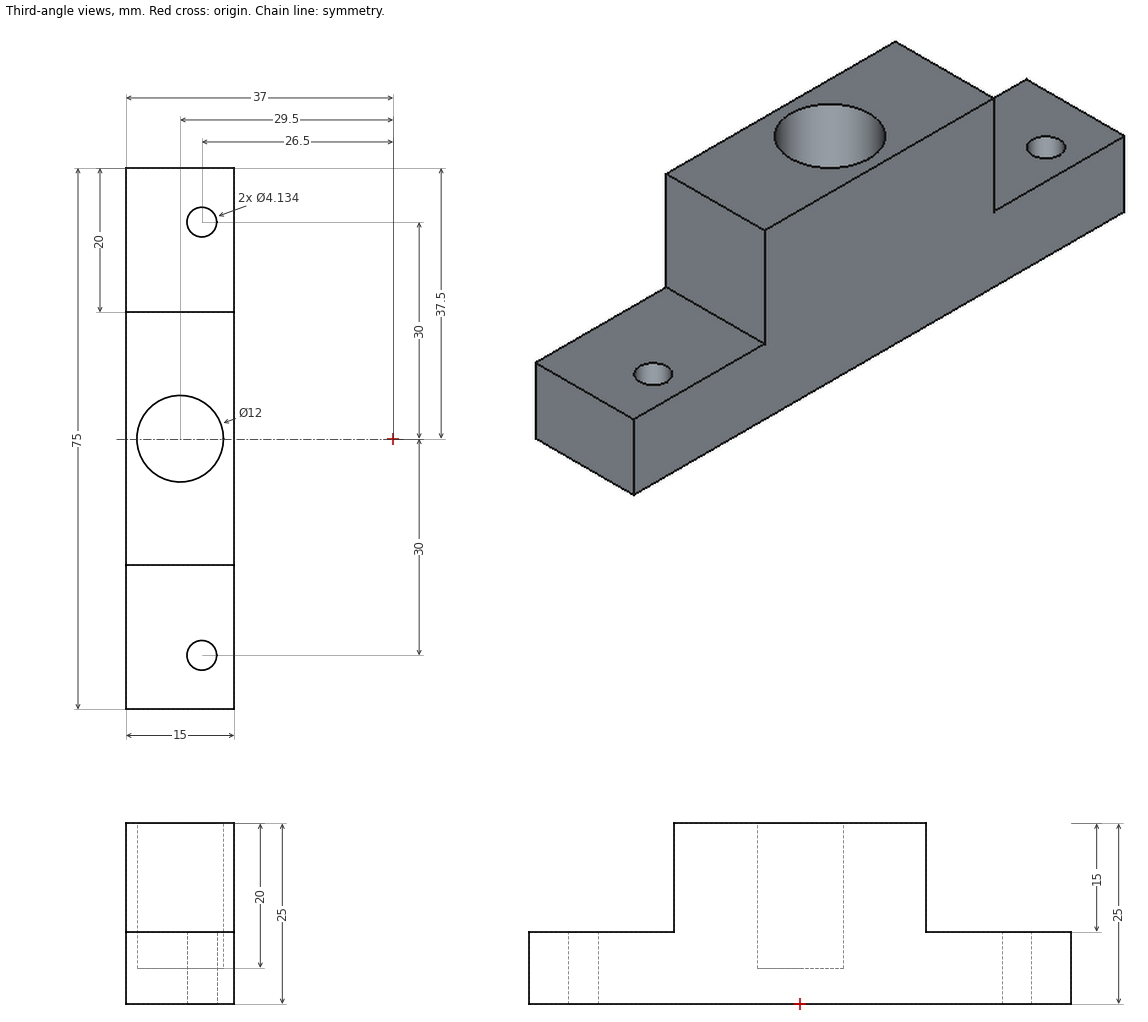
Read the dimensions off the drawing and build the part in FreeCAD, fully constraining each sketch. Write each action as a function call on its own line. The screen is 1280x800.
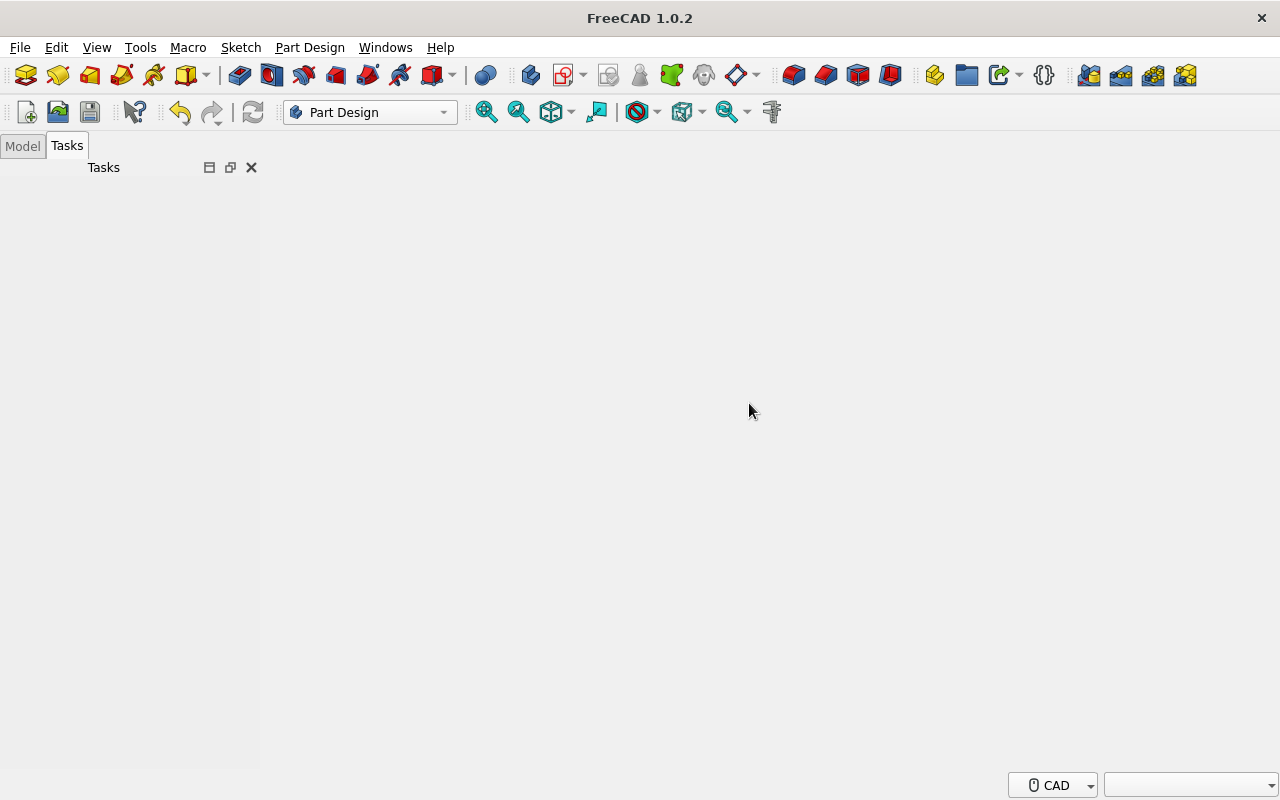
click(26, 112)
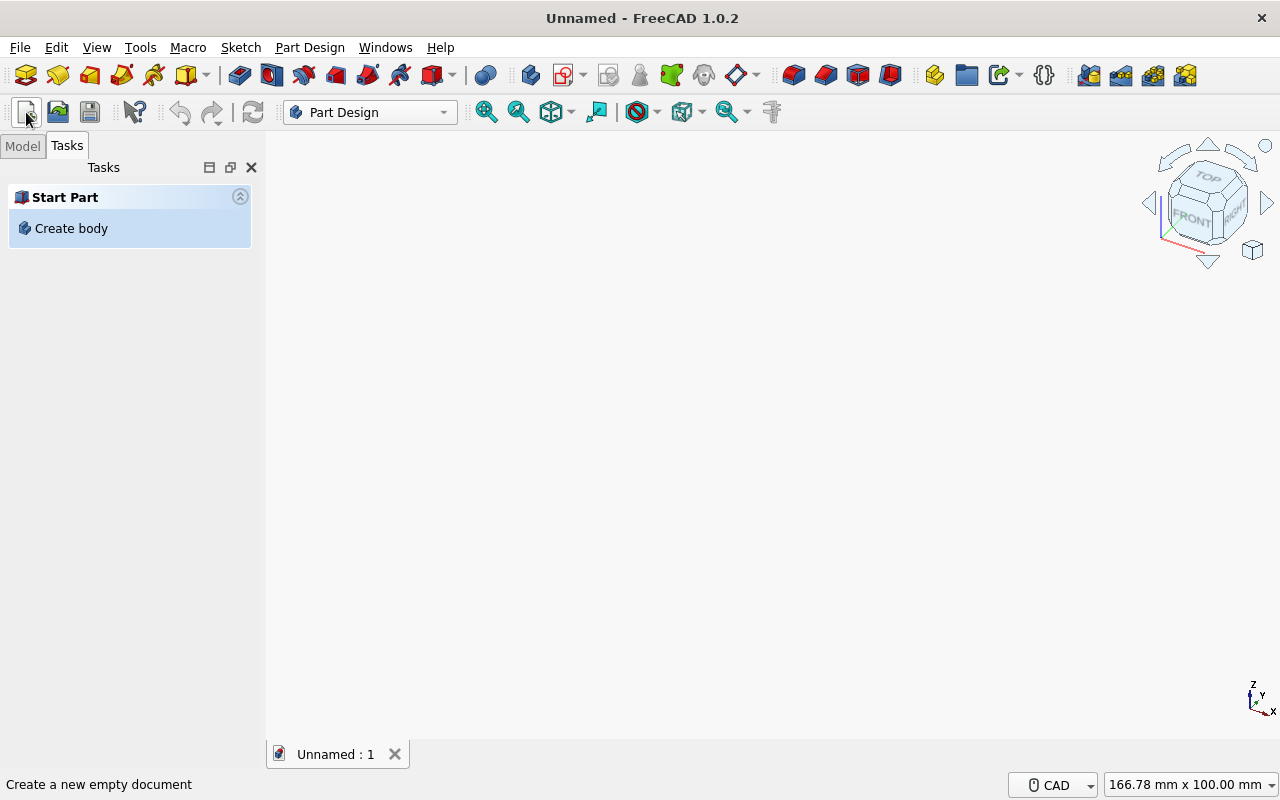
click(564, 76)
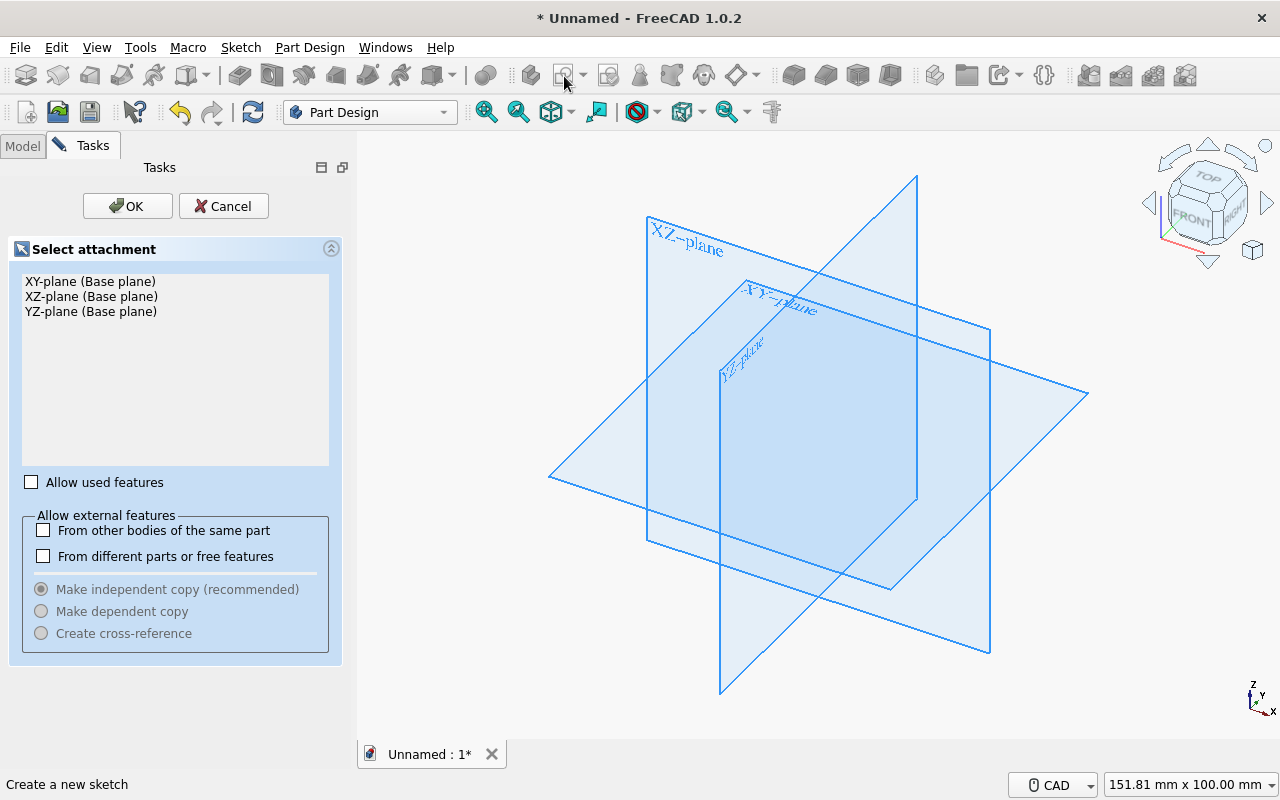
click(82, 282)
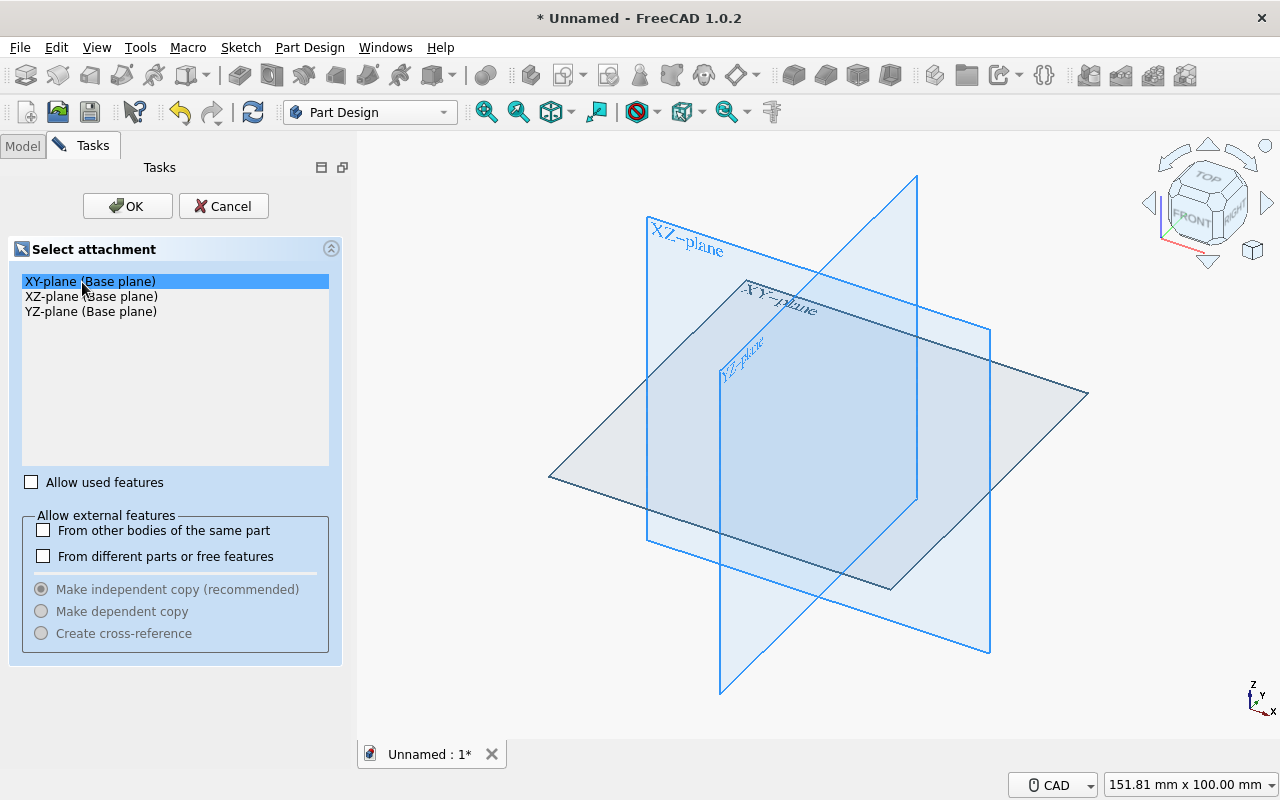
click(128, 206)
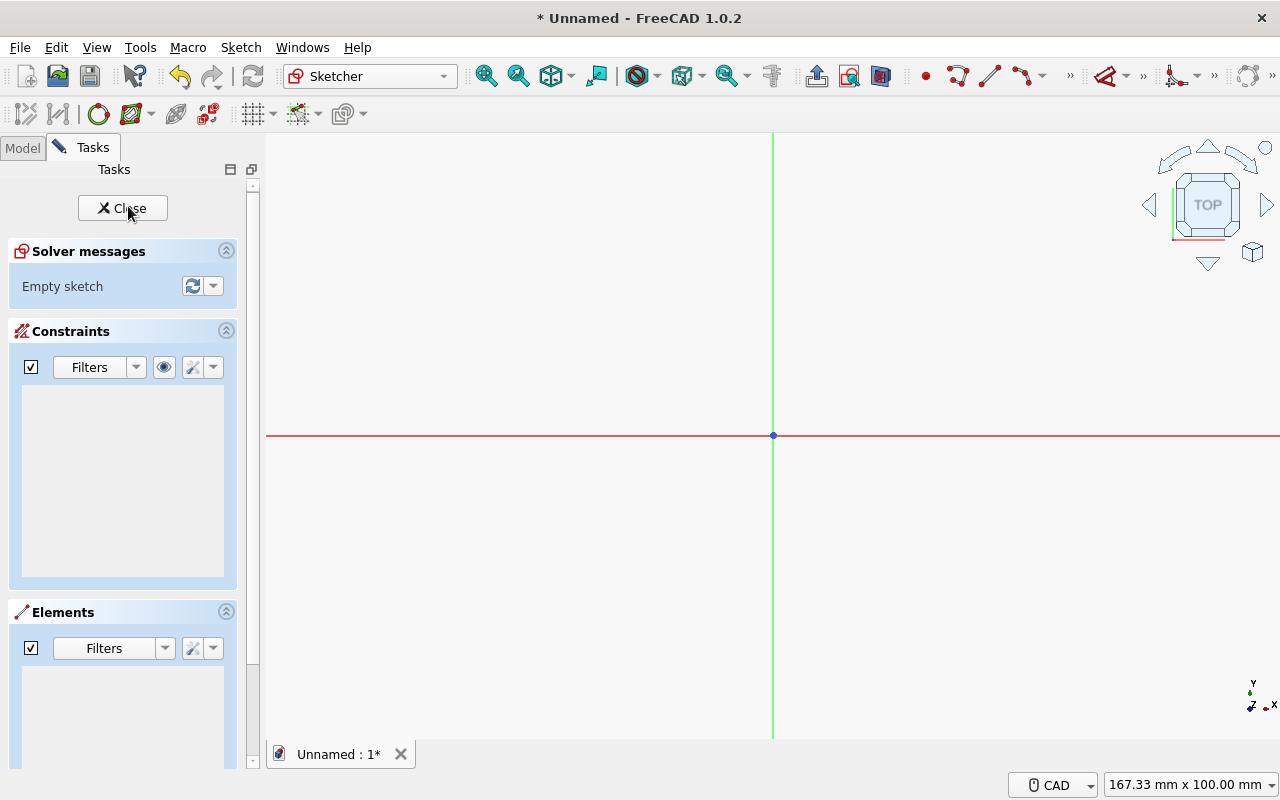
key(g)
key(r)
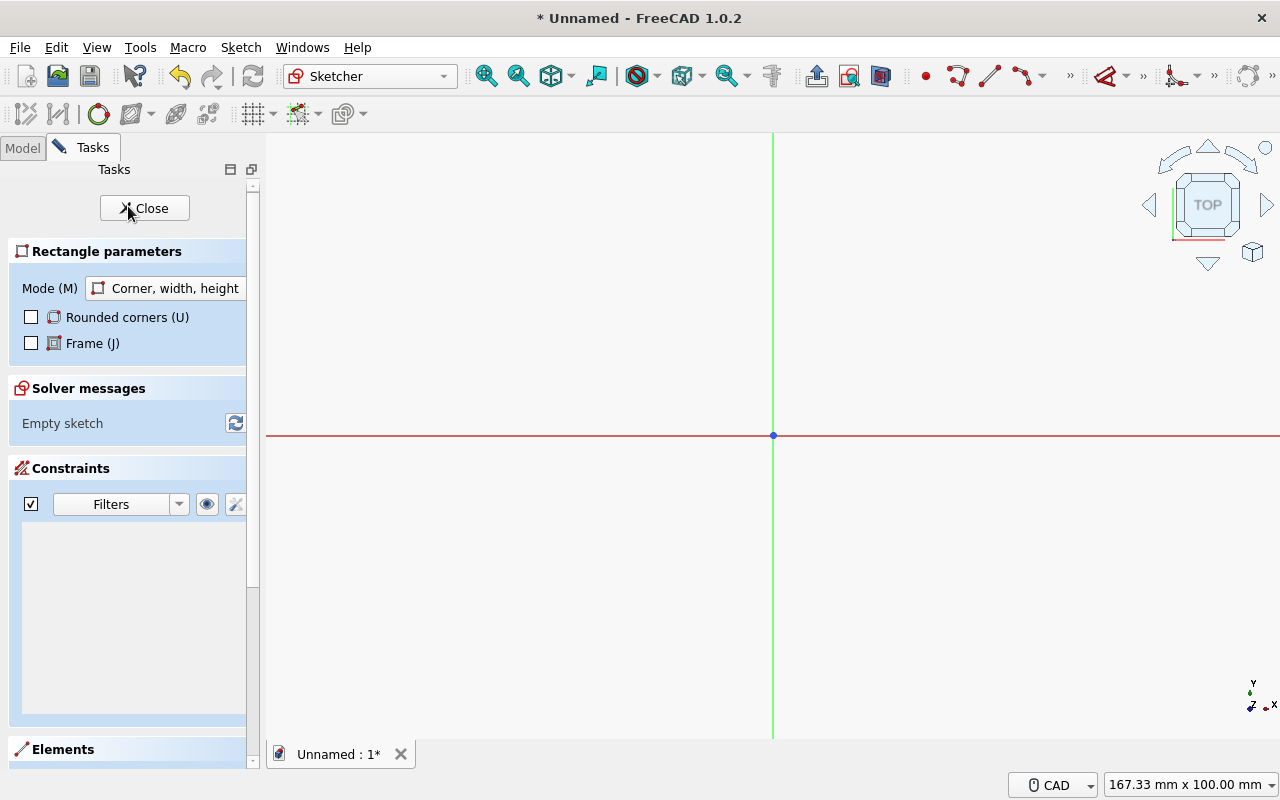
click(549, 209)
click(640, 663)
key(Escape)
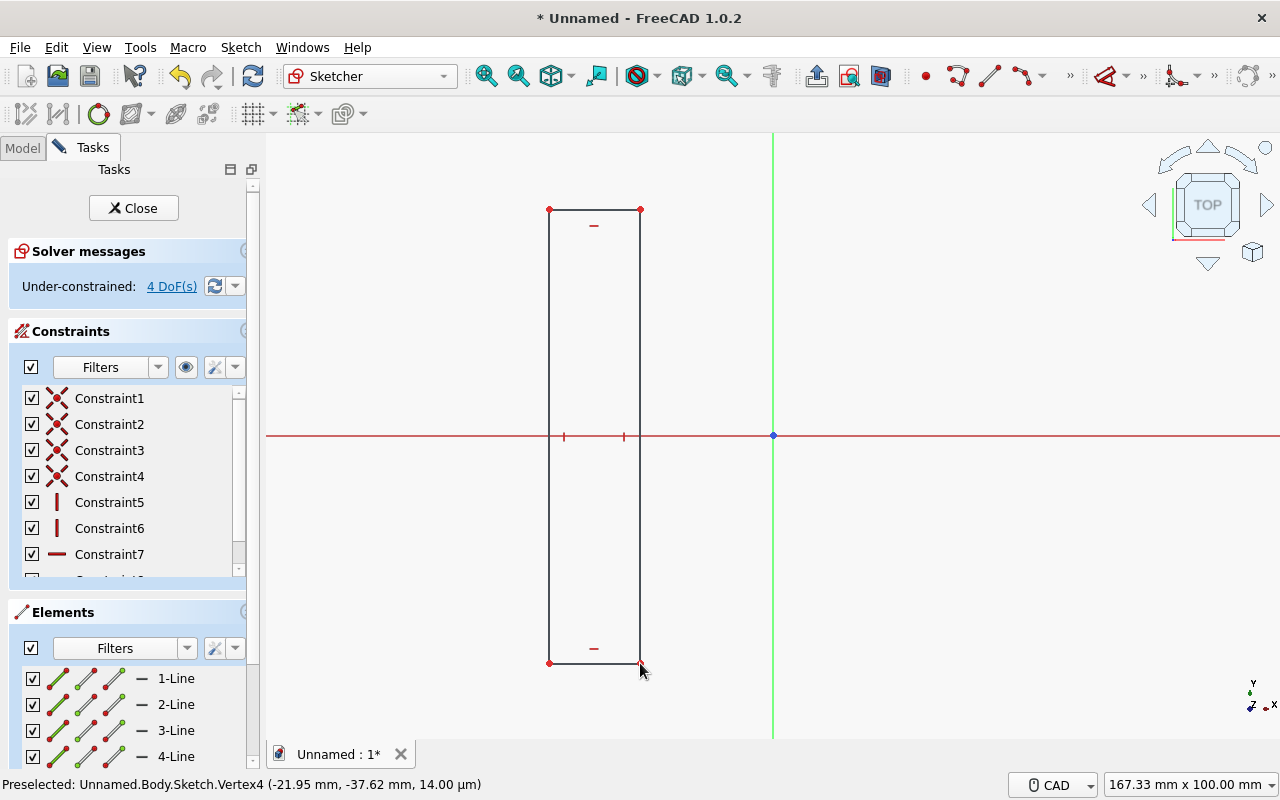
click(549, 346)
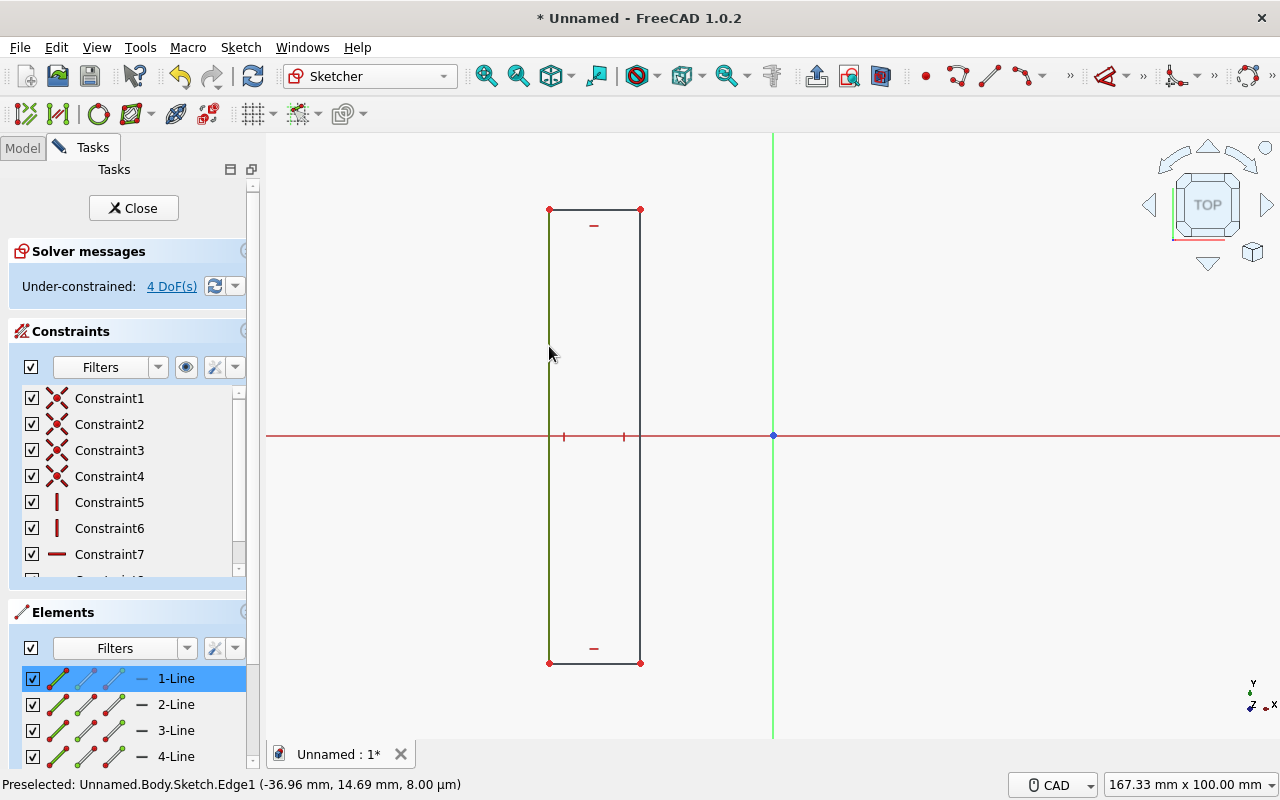
click(1128, 76)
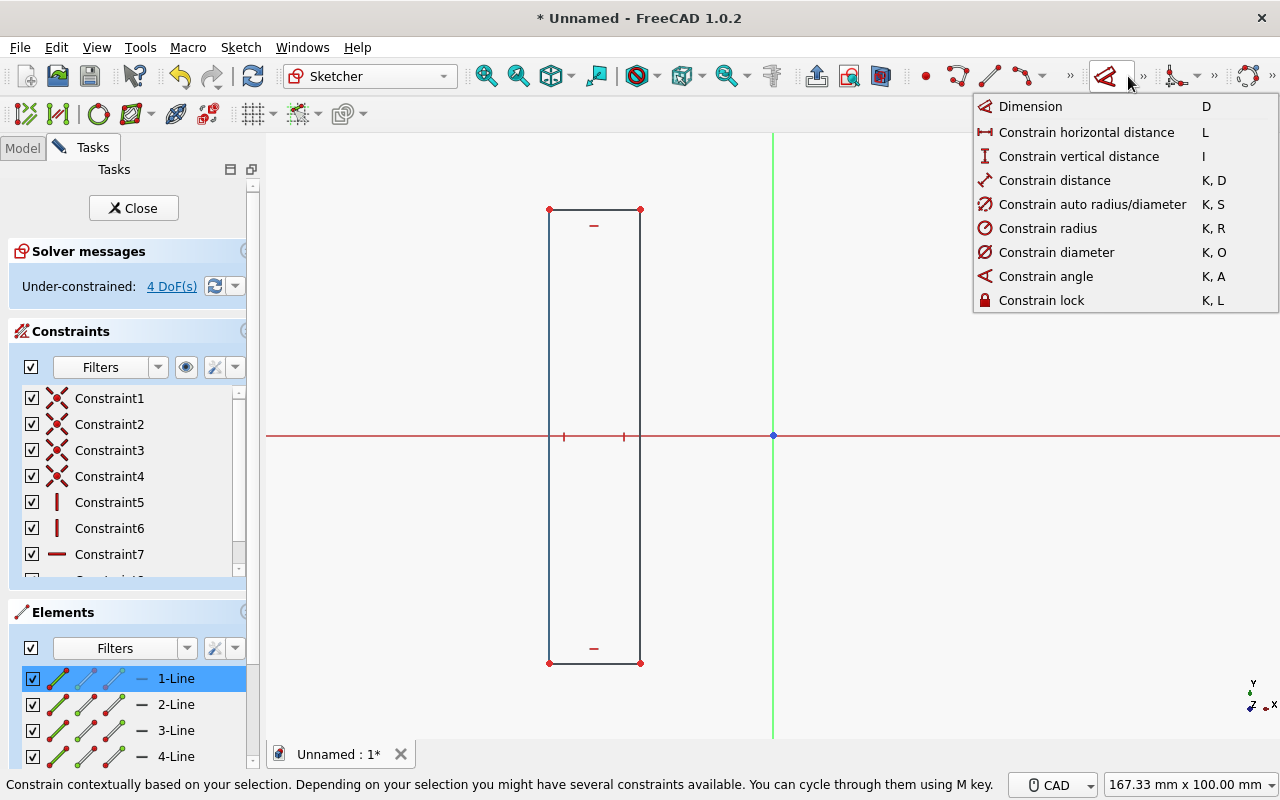
click(1126, 156)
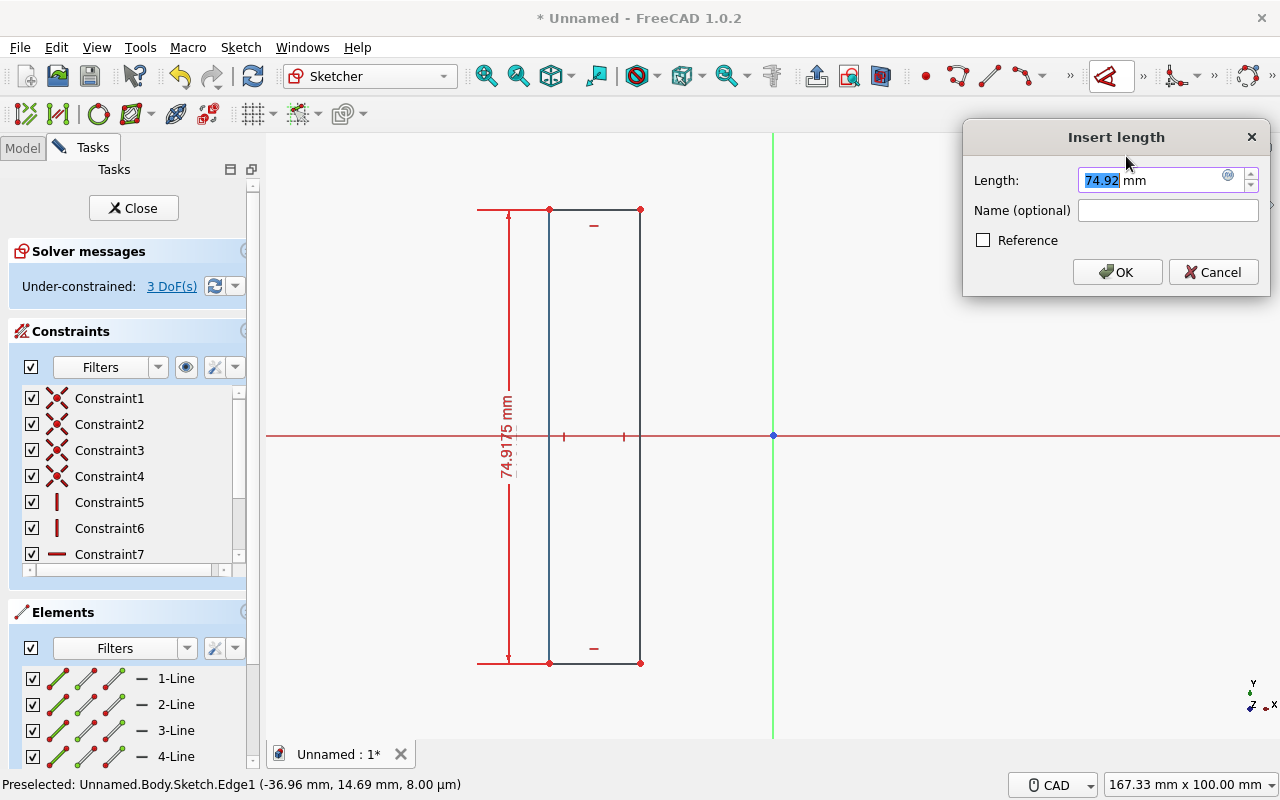
text(75)
key(Return)